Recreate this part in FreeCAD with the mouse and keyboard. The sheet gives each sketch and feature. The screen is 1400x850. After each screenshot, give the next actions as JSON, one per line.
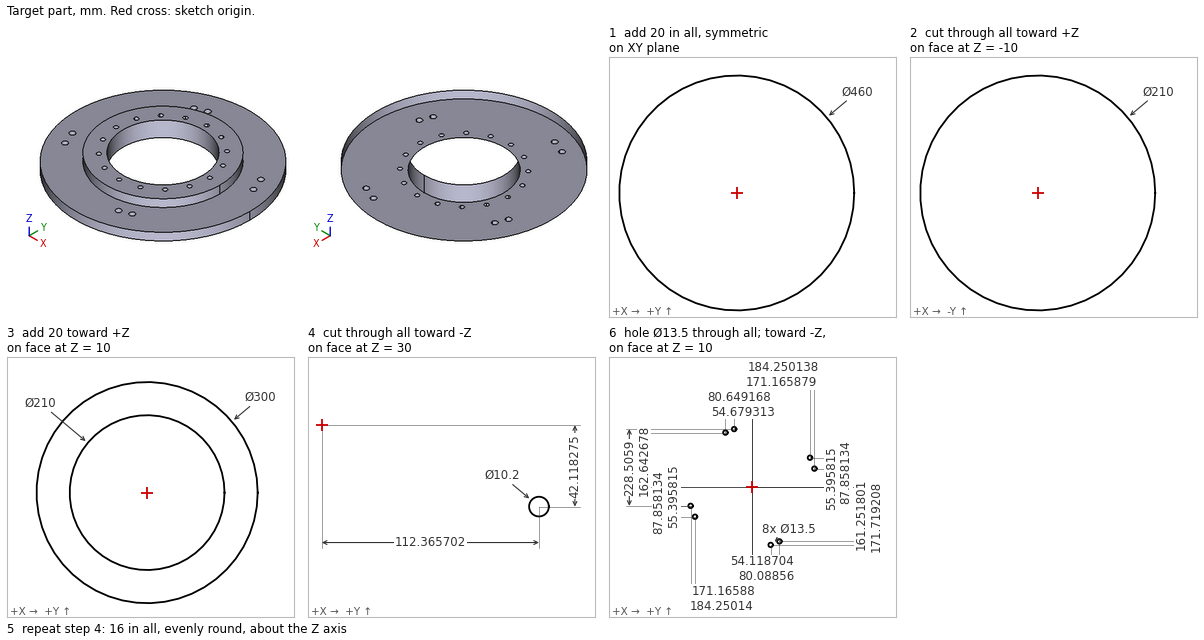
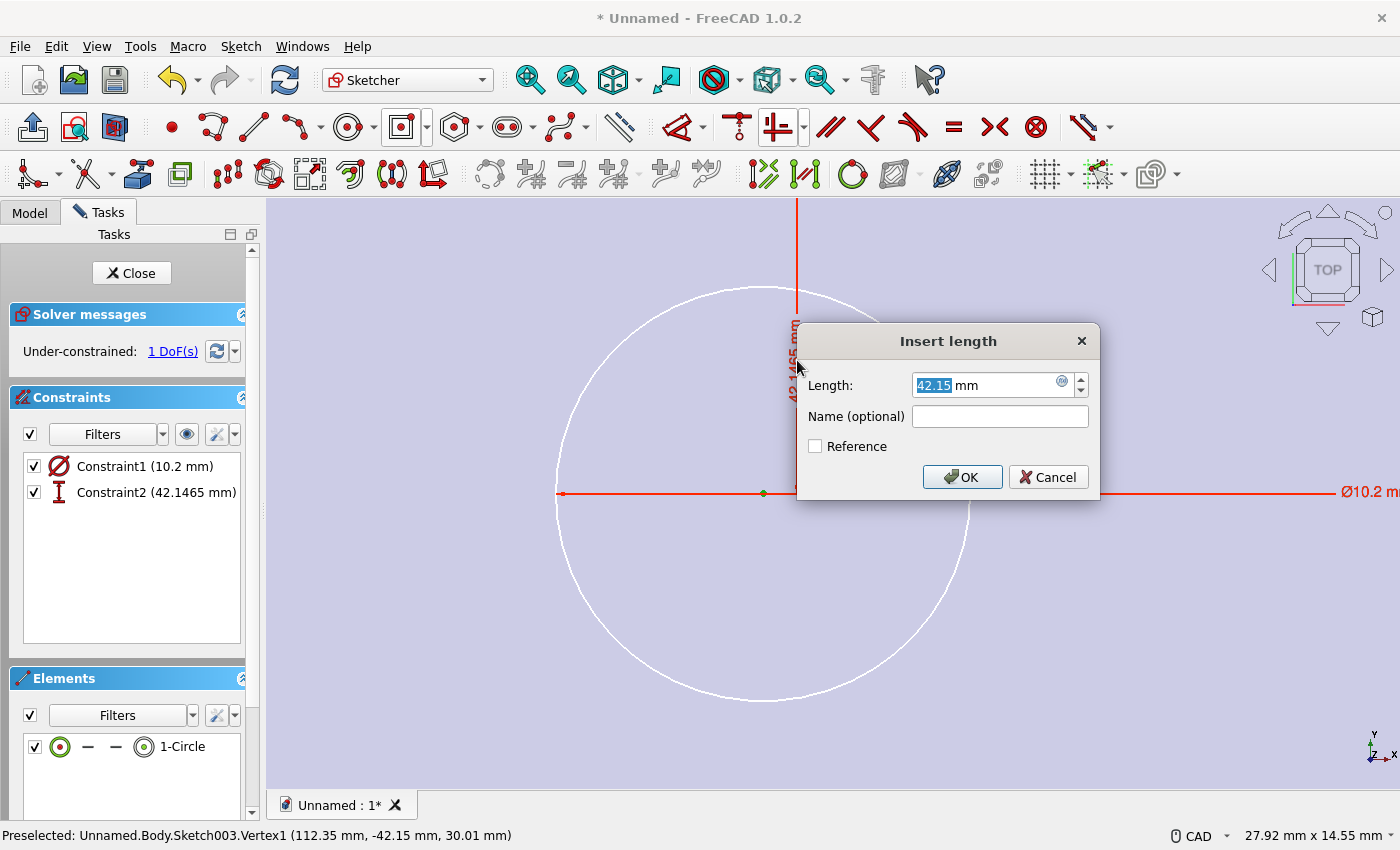
{"action": "type", "text": "42.118275"}
{"action": "key", "text": "Return"}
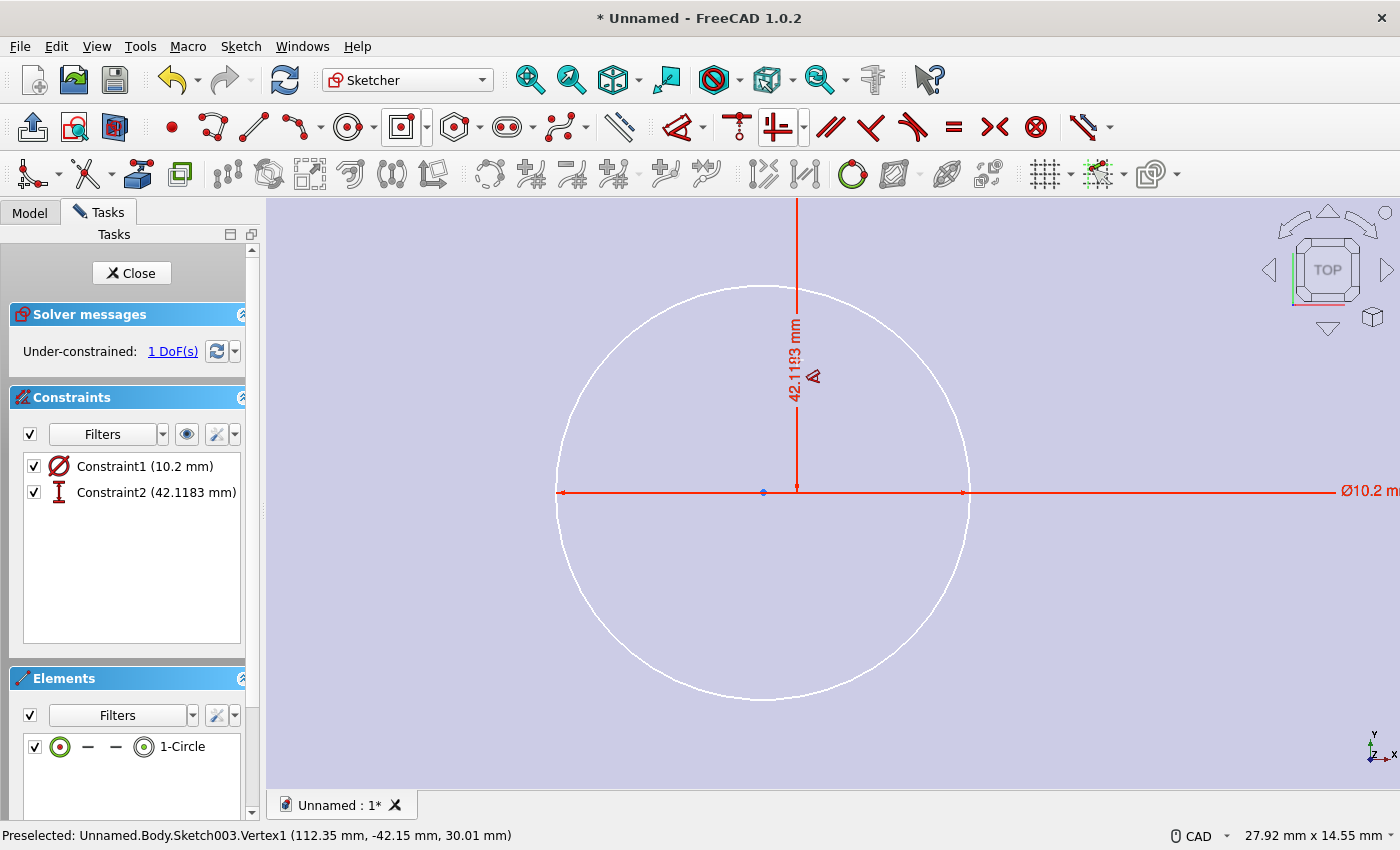
{"action": "left_click", "coordinate": [763, 493]}
{"action": "left_click", "coordinate": [528, 527]}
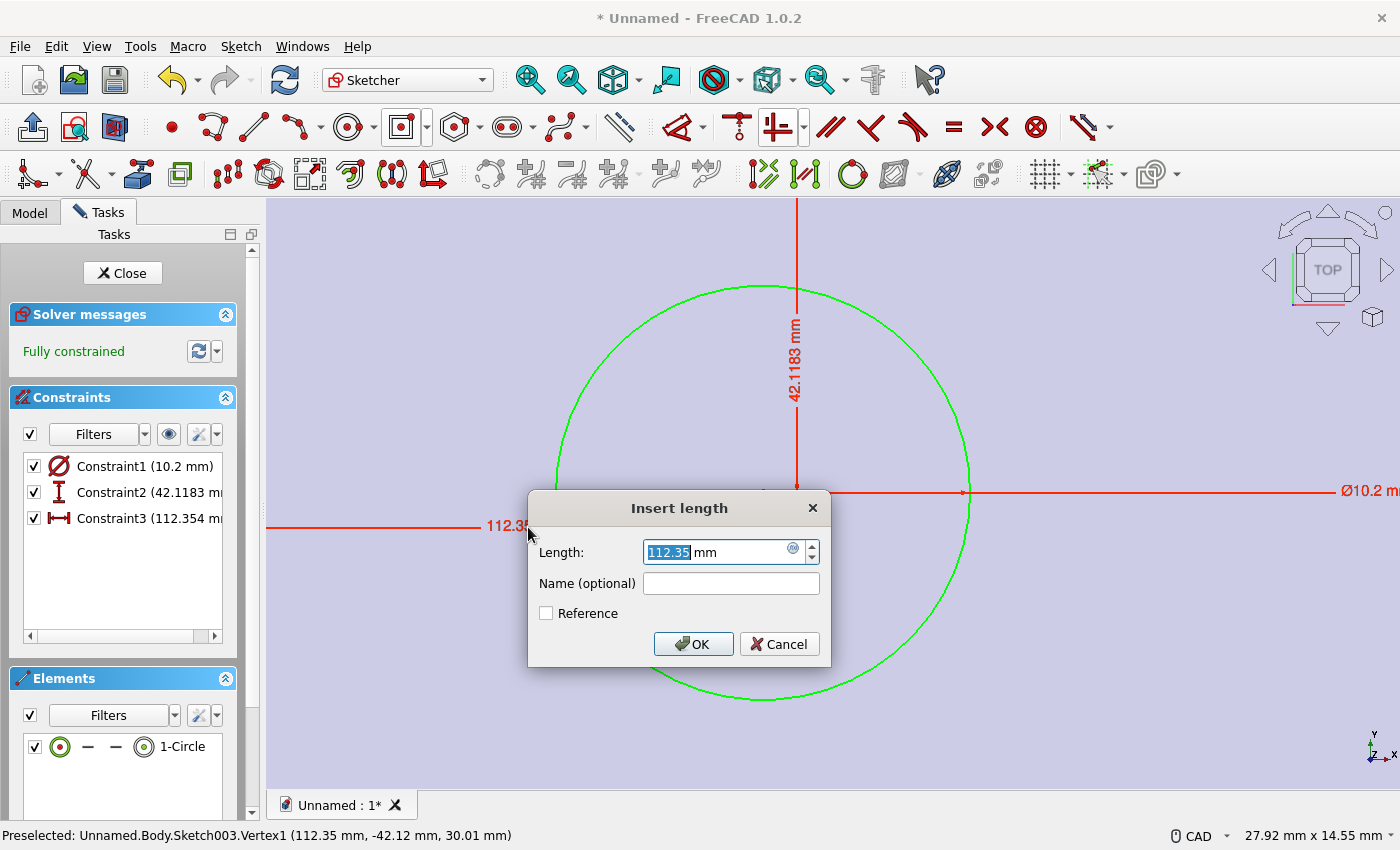
{"action": "type", "text": "112.365702"}
{"action": "key", "text": "Return"}
{"action": "key", "text": "Escape"}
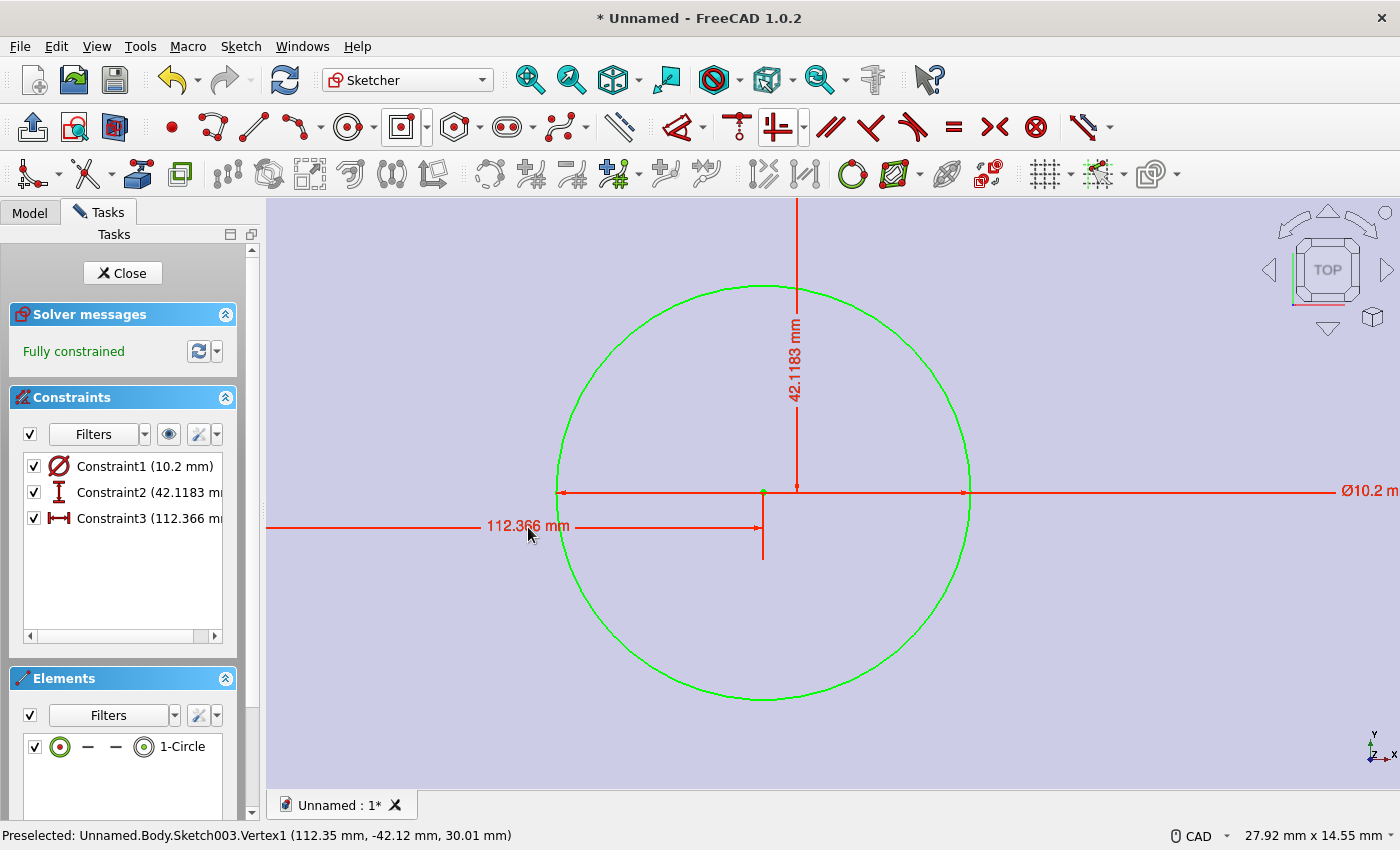
{"action": "left_click", "coordinate": [123, 273]}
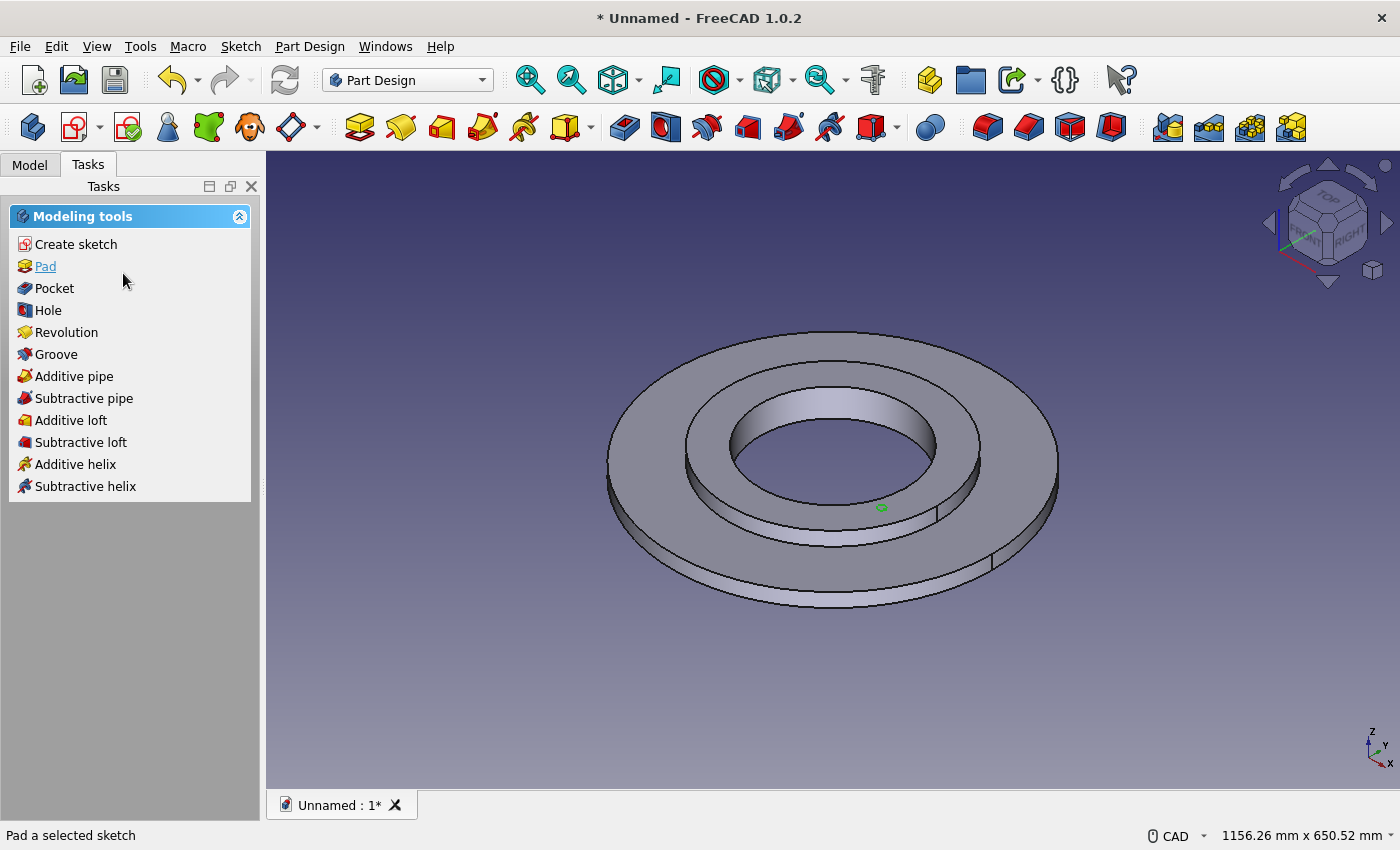
{"action": "left_click", "coordinate": [625, 128]}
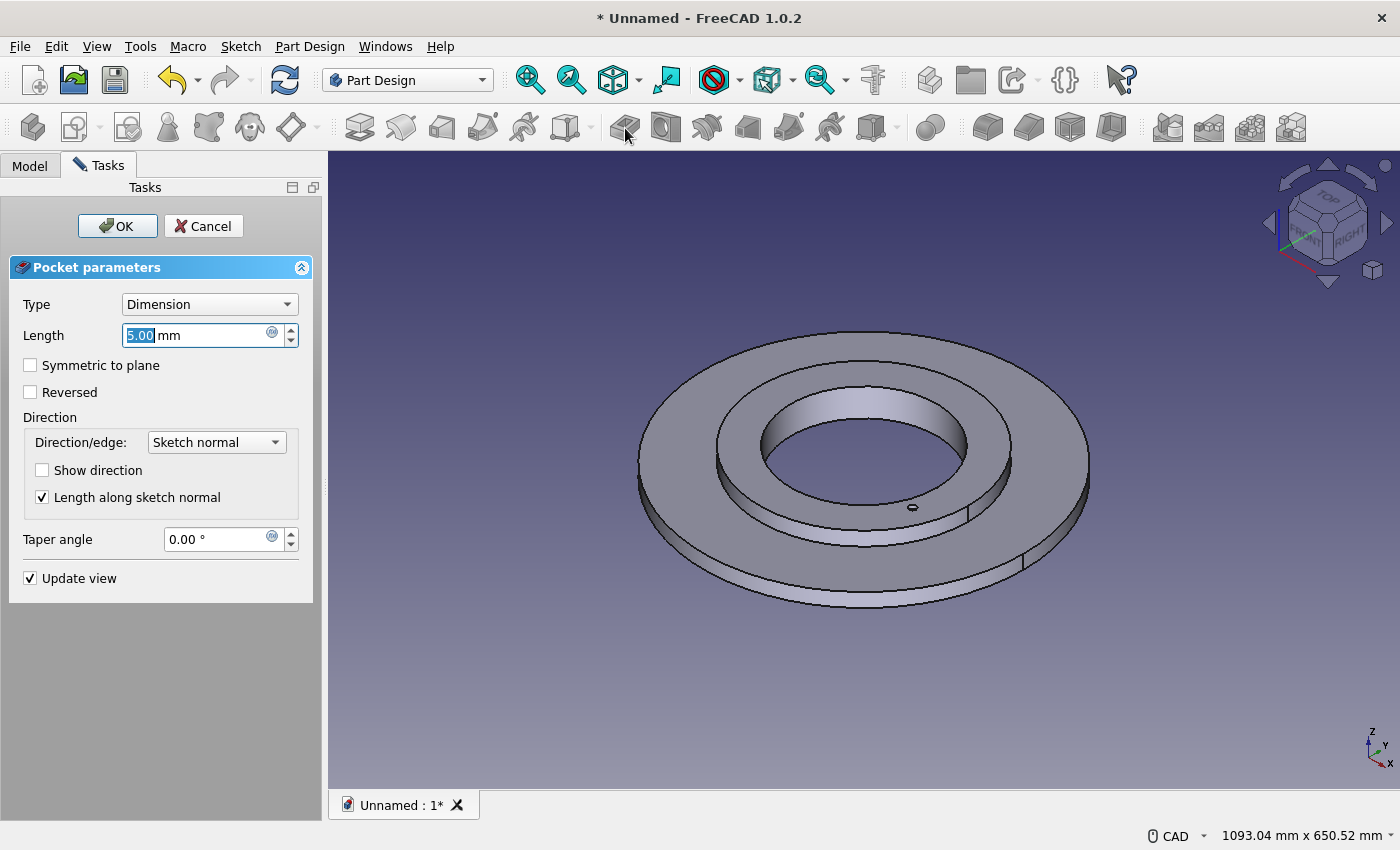
{"action": "left_click", "coordinate": [210, 304]}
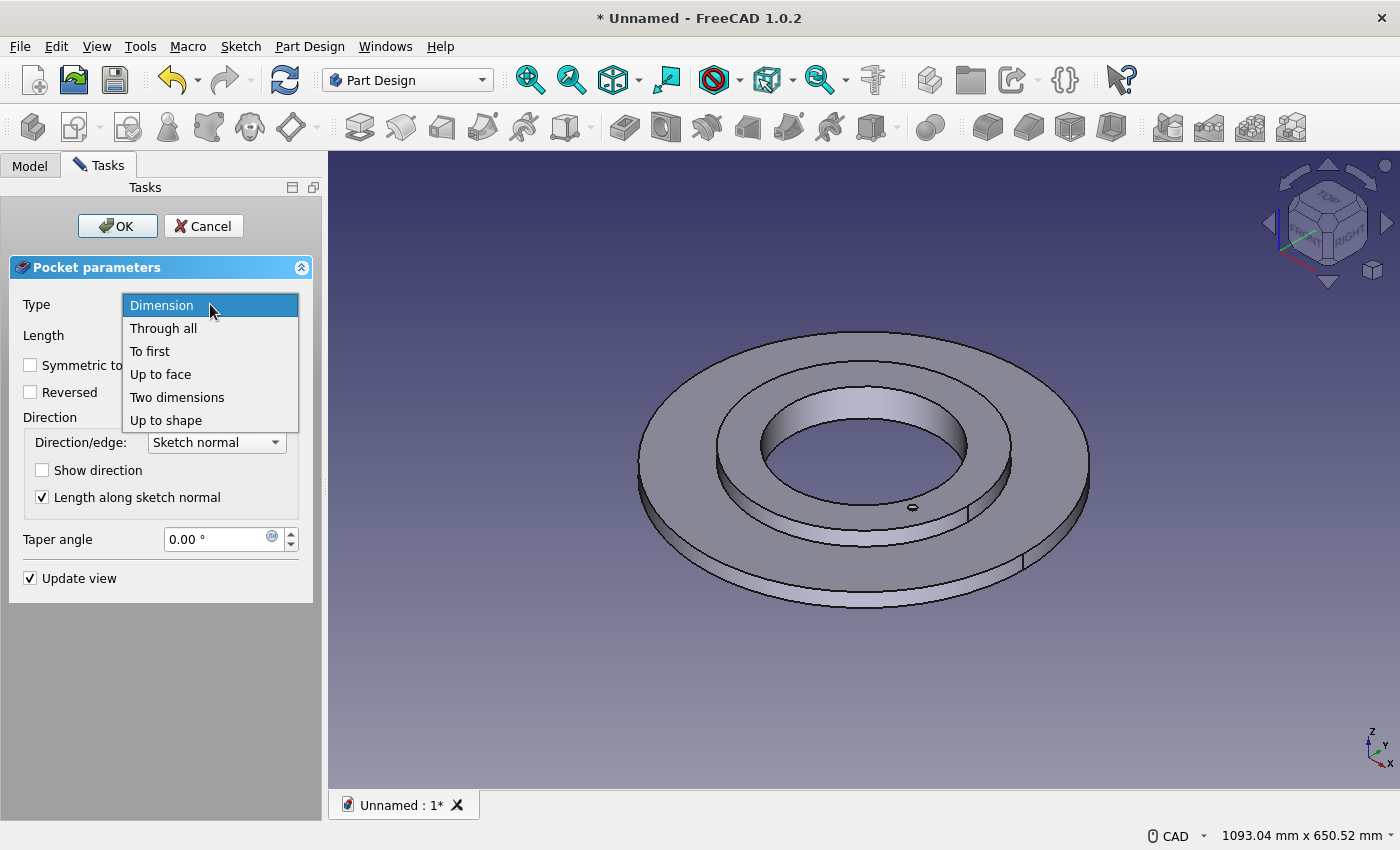
{"action": "left_click", "coordinate": [208, 328]}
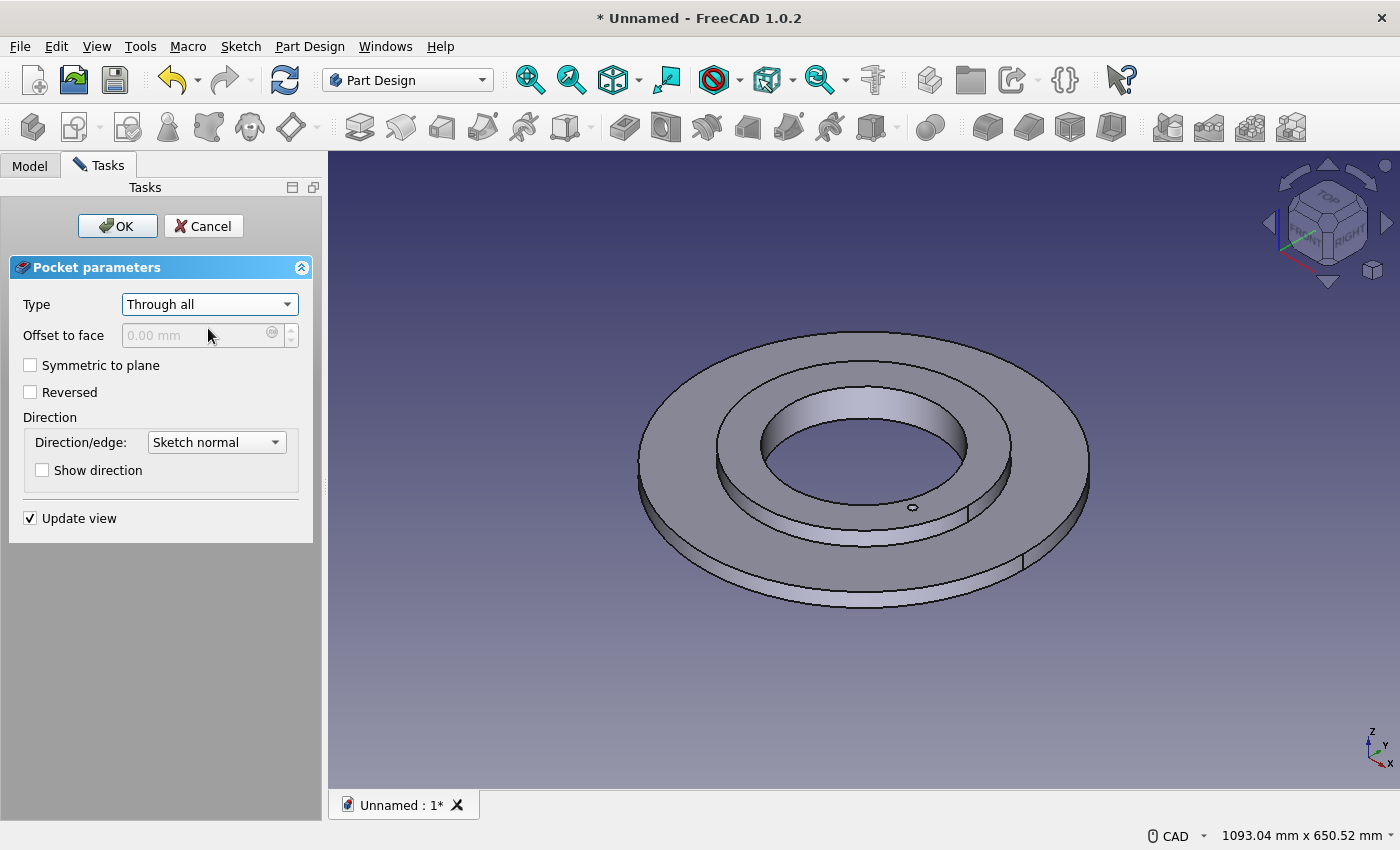
{"action": "left_click", "coordinate": [118, 226]}